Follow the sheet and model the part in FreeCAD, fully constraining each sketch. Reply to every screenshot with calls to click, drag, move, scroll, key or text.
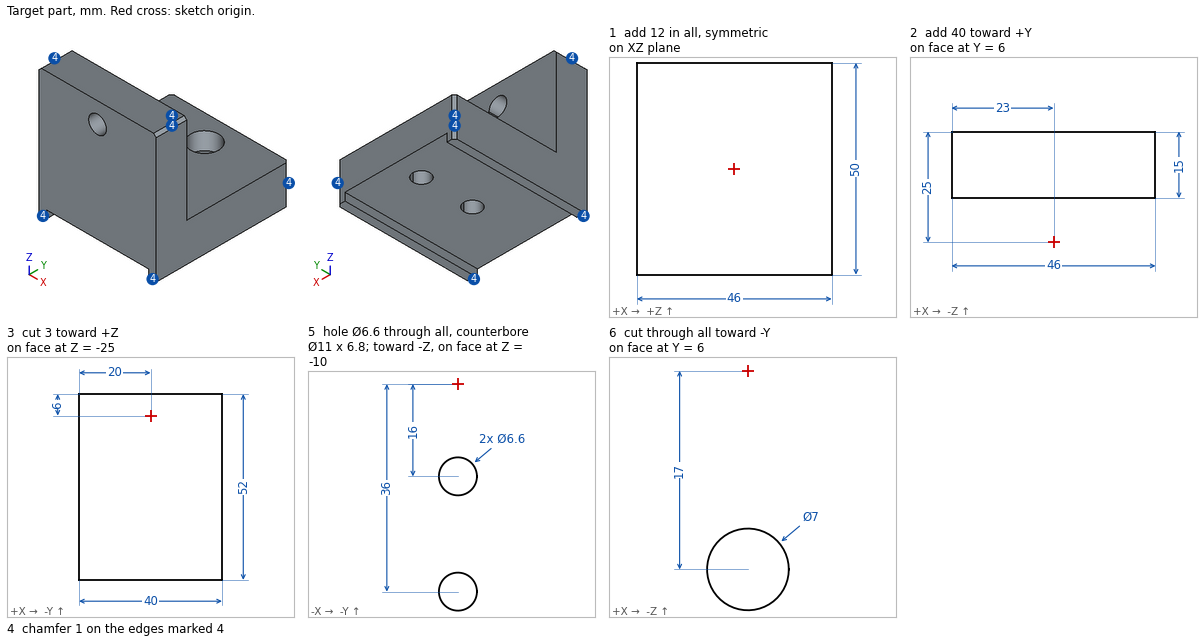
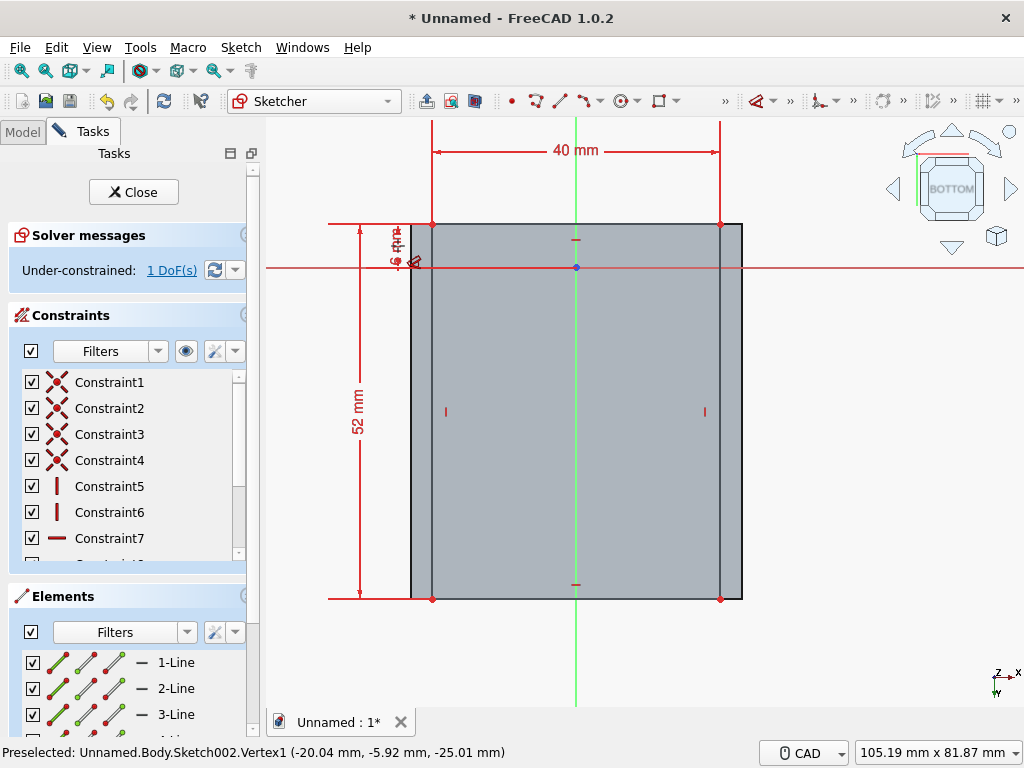
click(432, 224)
click(504, 190)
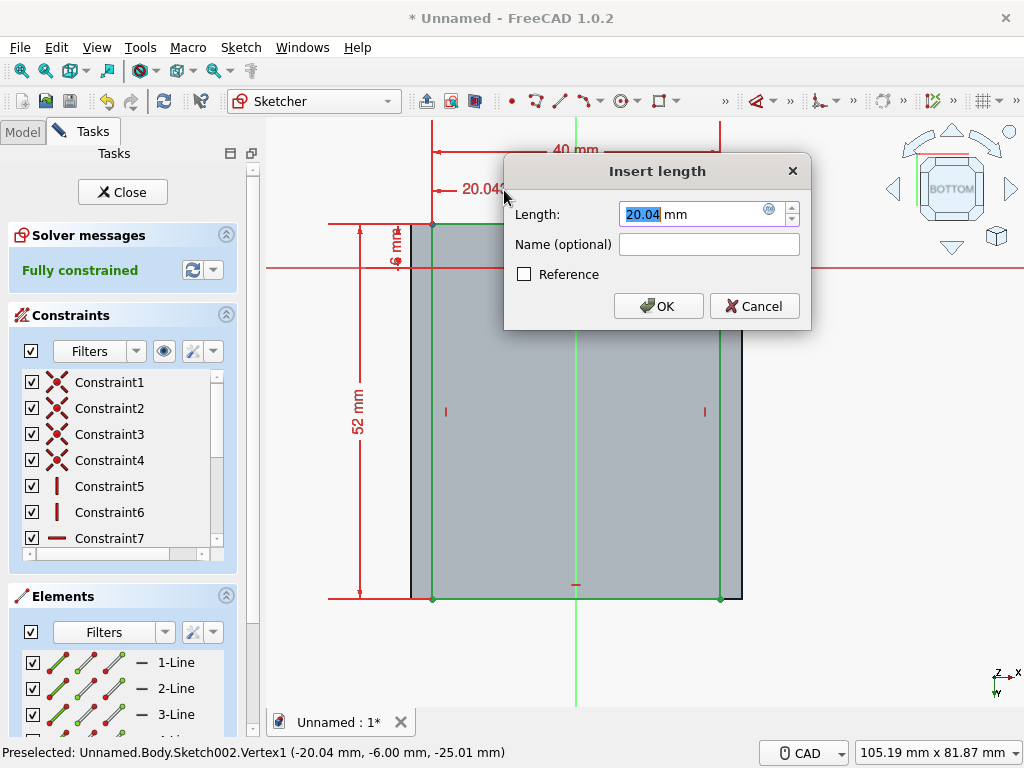
text(20)
key(Return)
key(Escape)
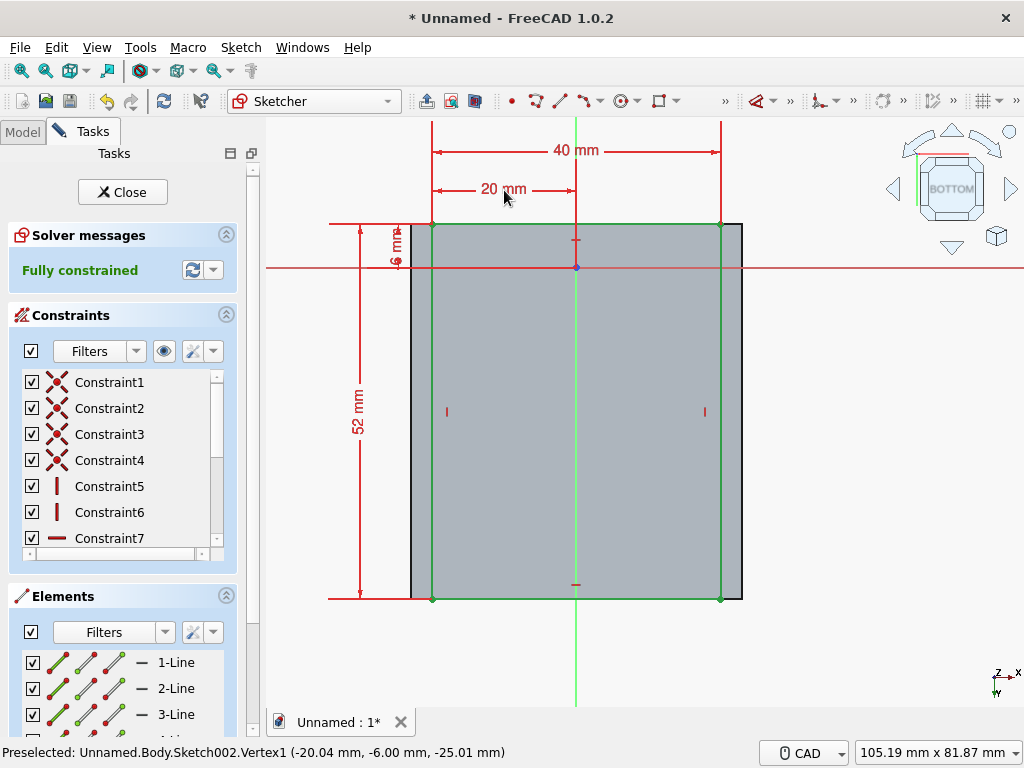
click(123, 192)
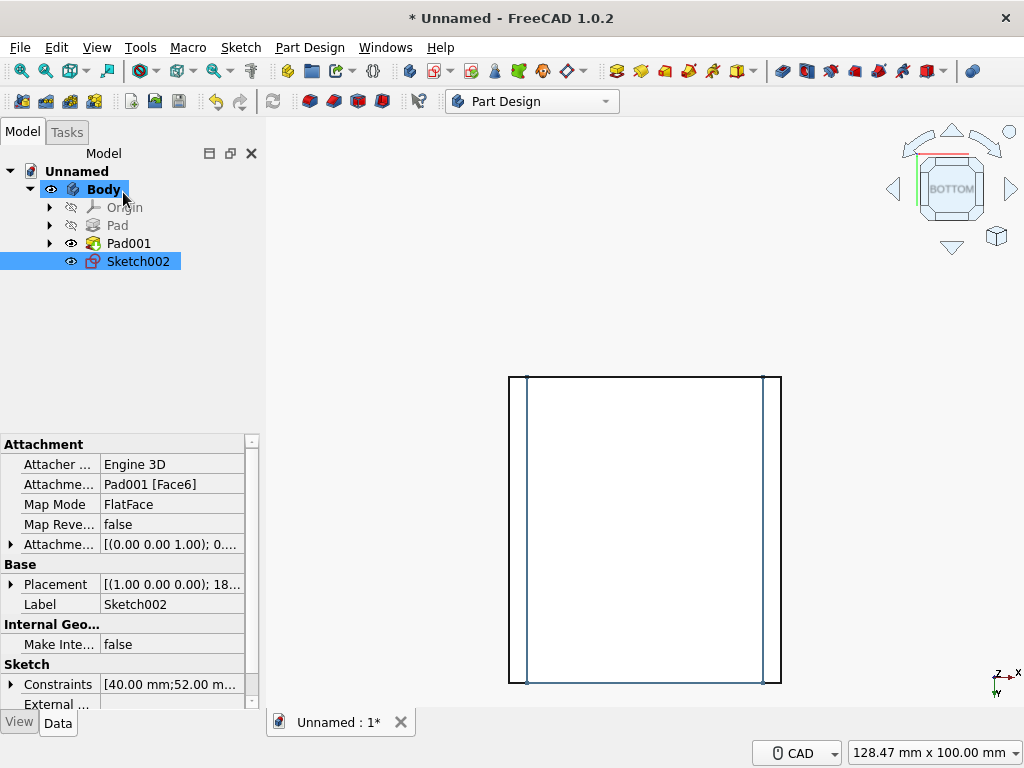
click(784, 72)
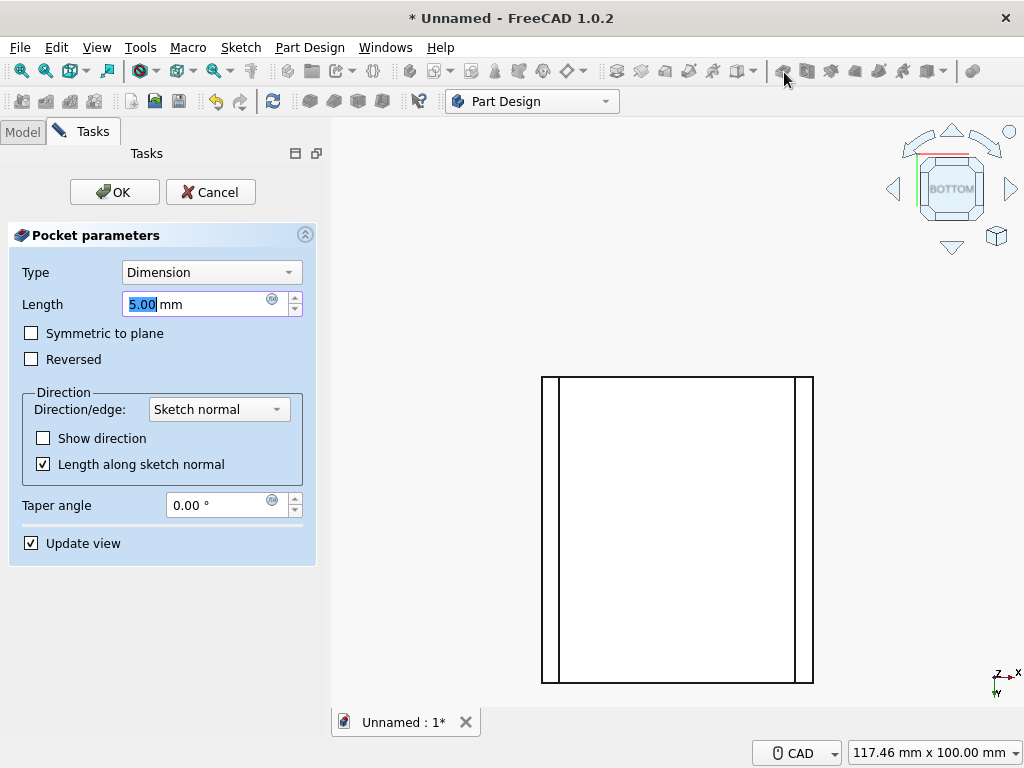
text(3)
key(Tab)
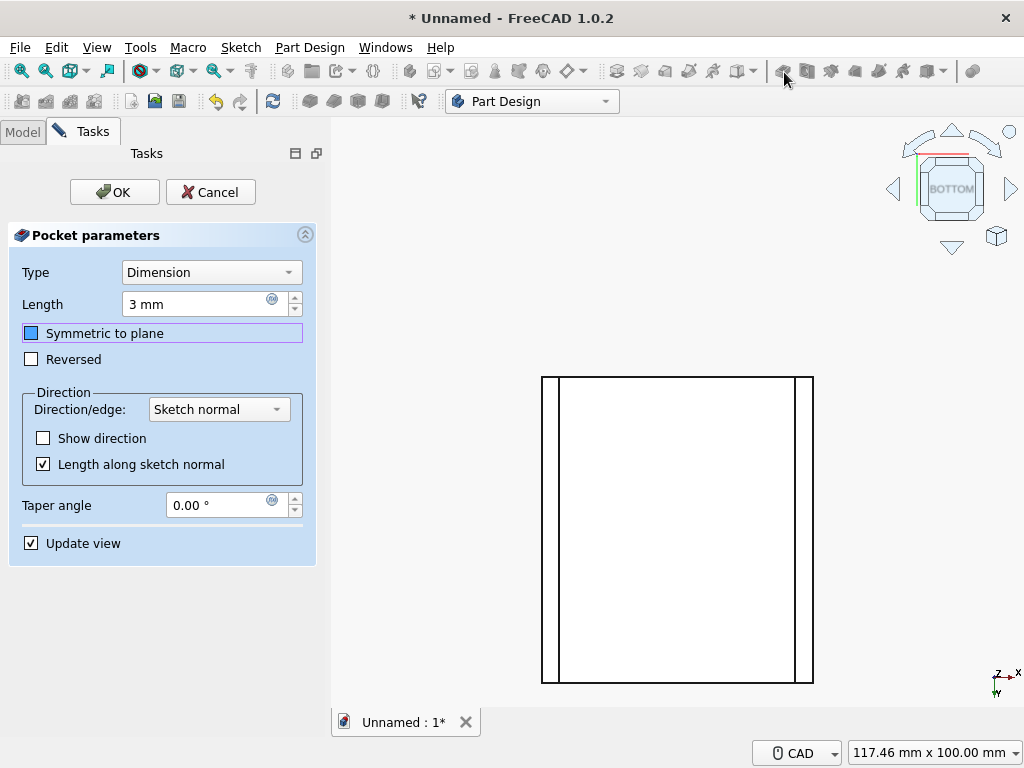
click(115, 192)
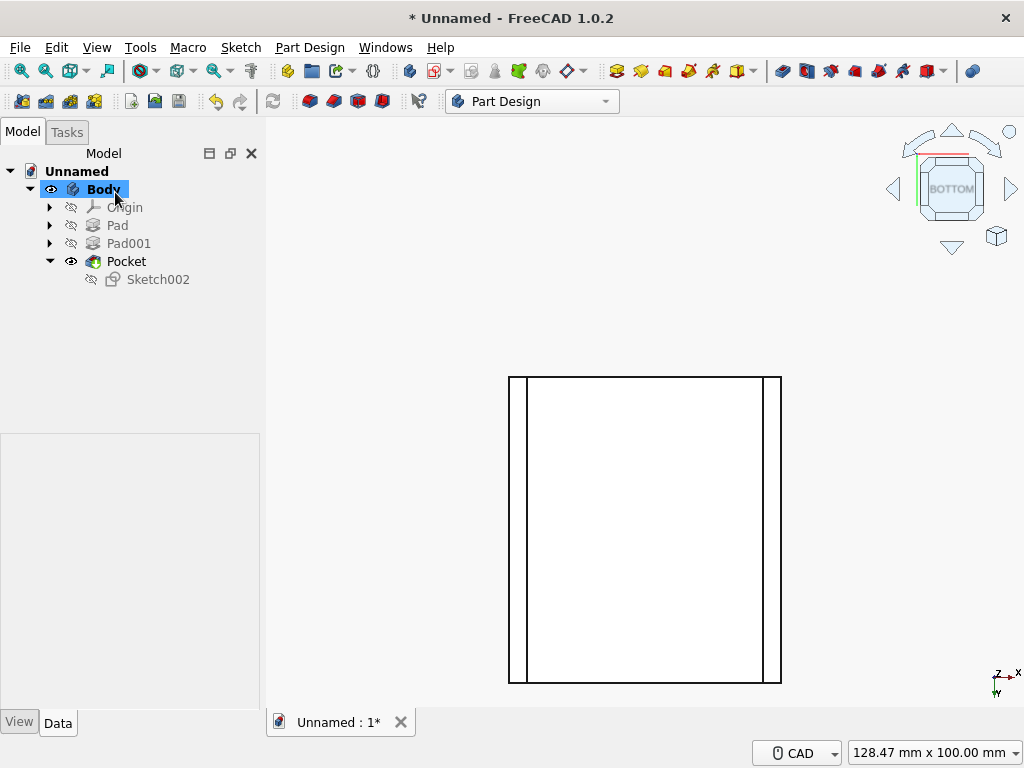
click(518, 376)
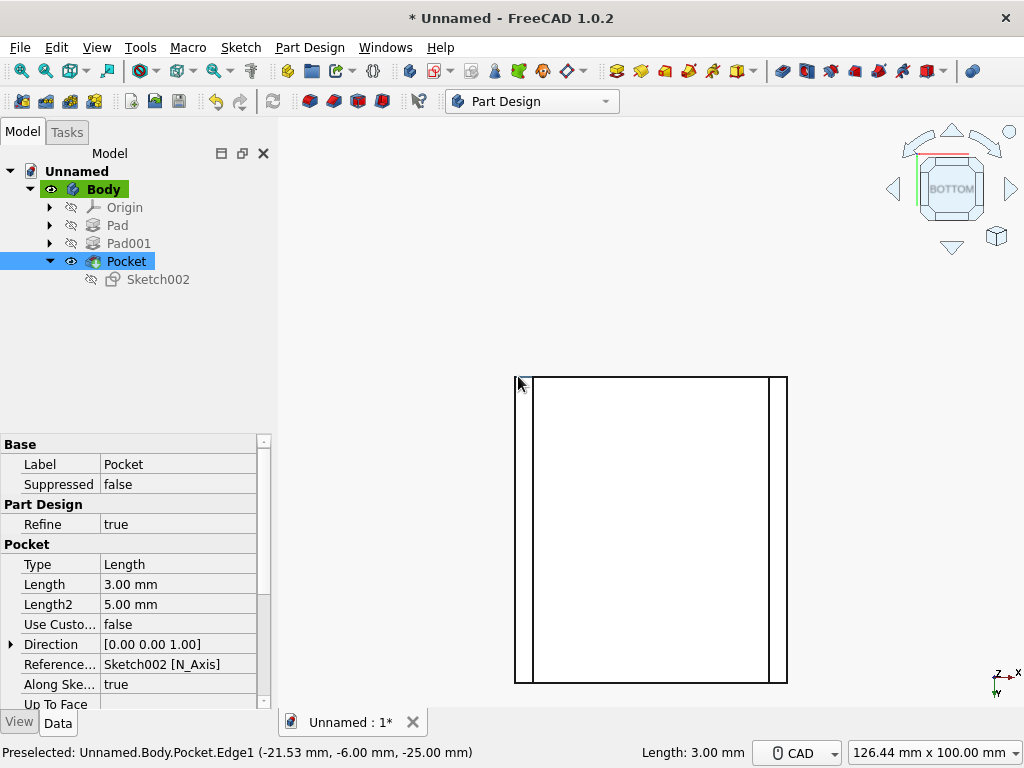
click(778, 376, ctrl)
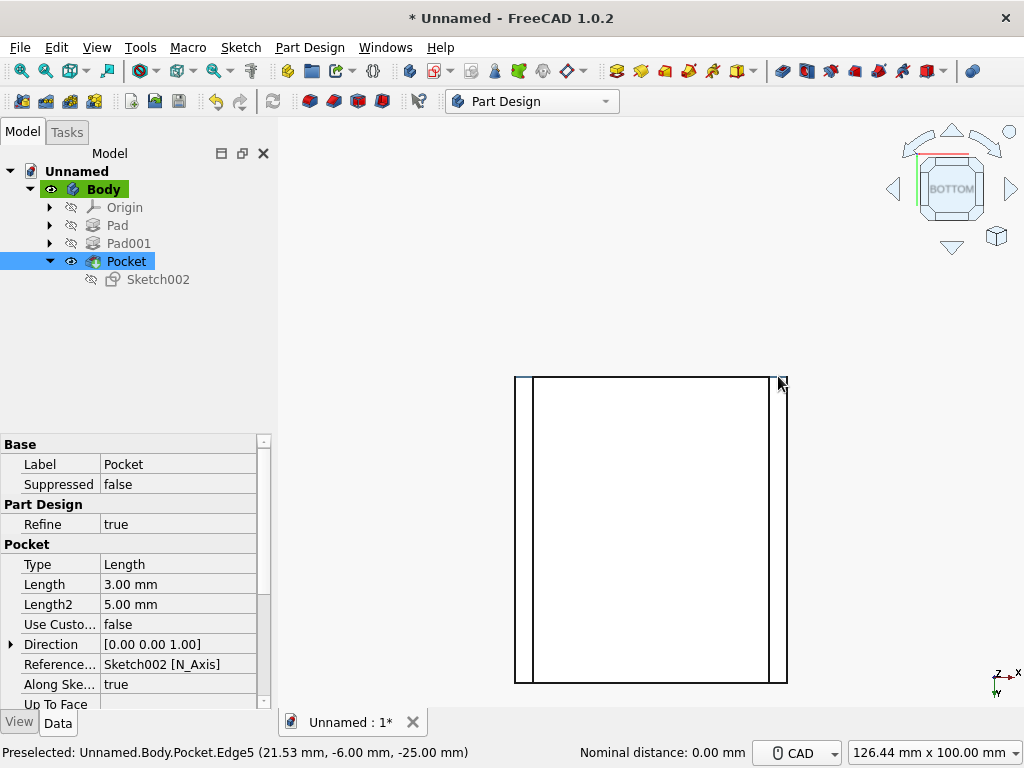
key(0)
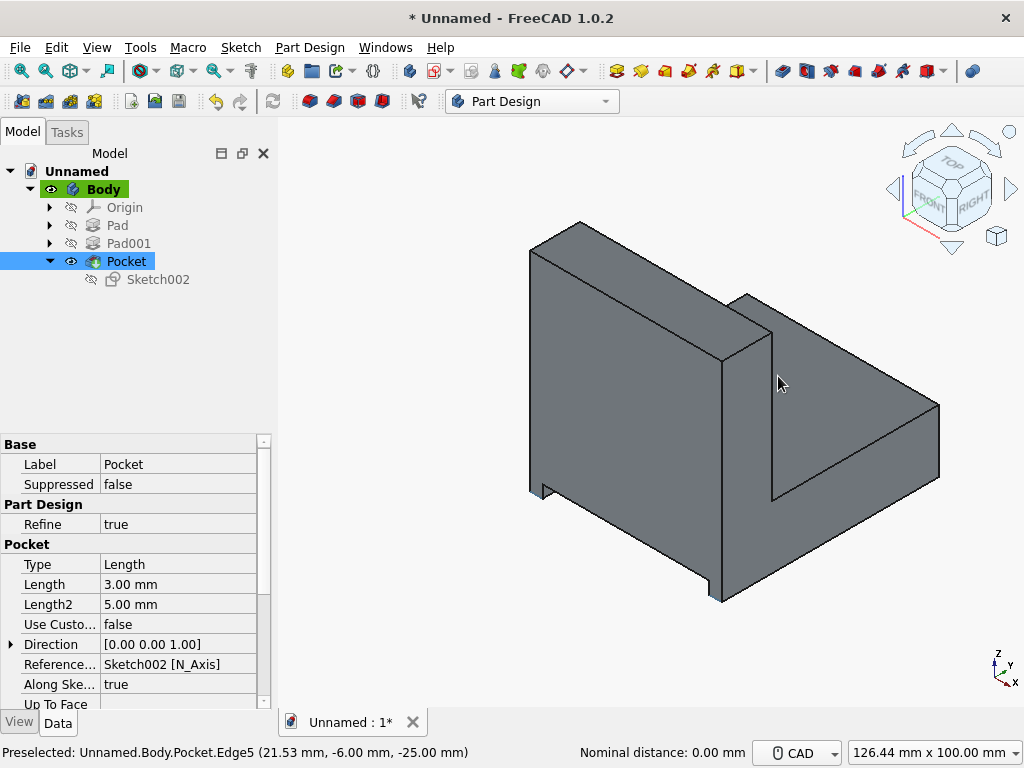
click(747, 346, ctrl)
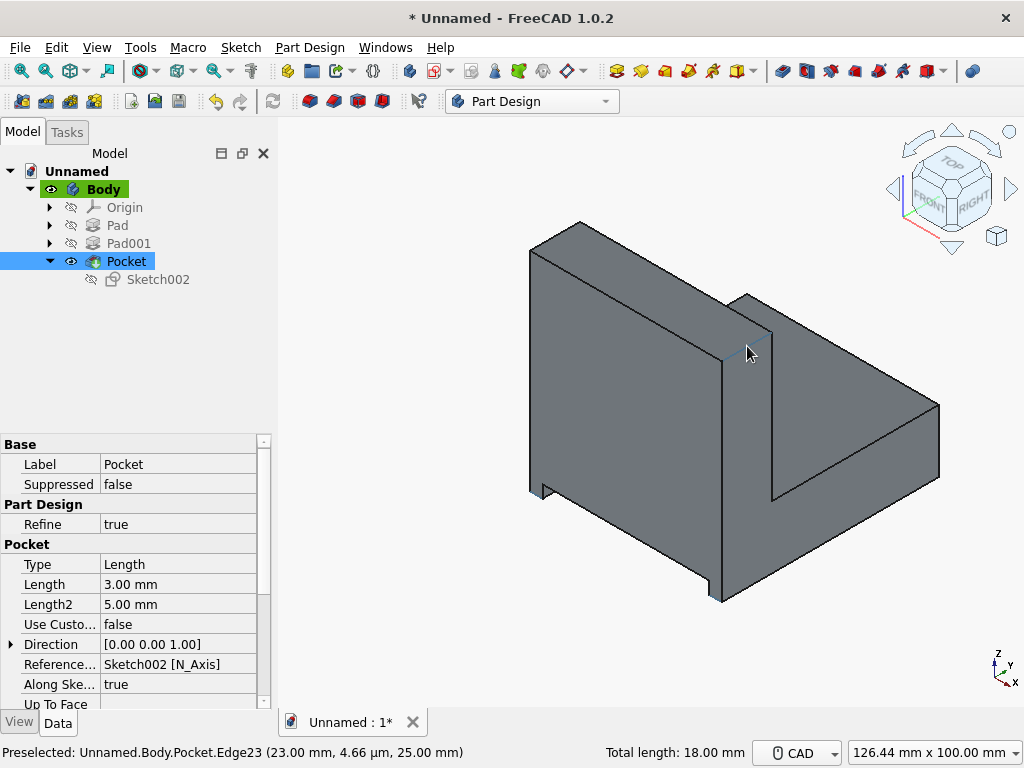
key(2)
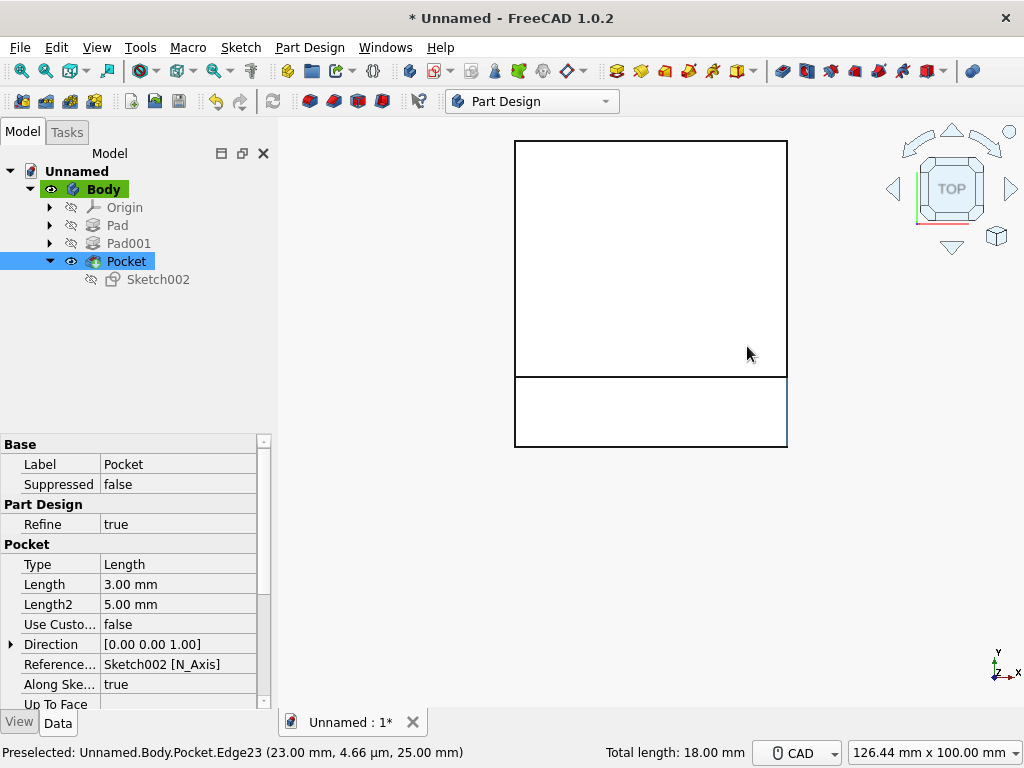
click(515, 411, ctrl)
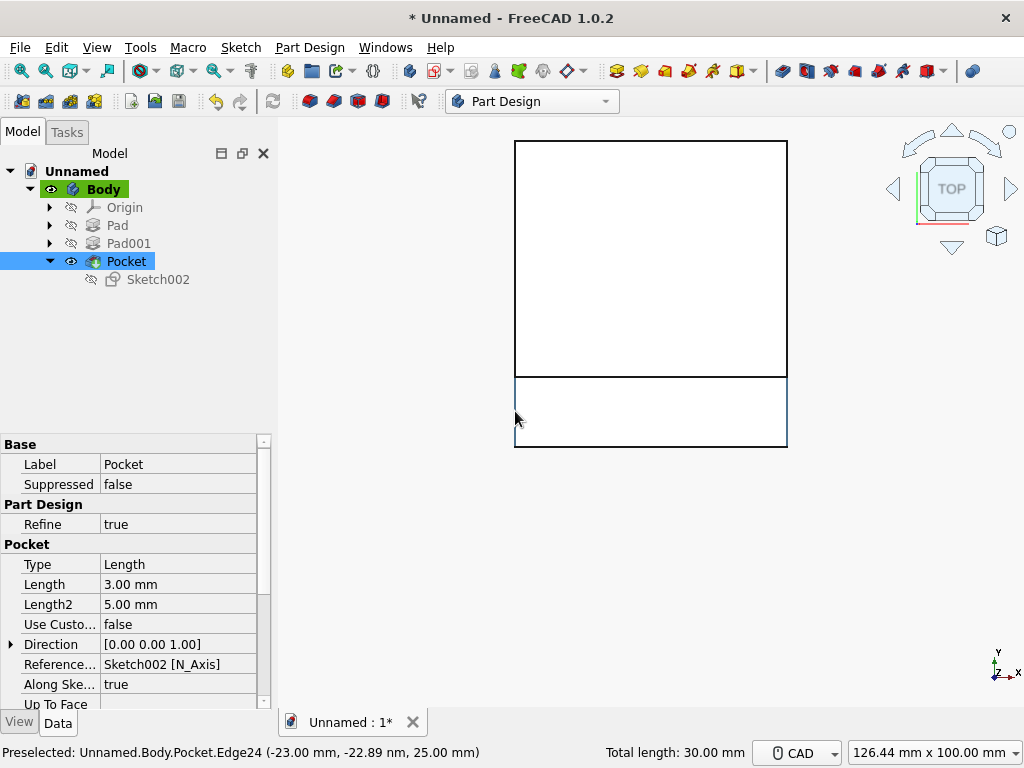
key(1)